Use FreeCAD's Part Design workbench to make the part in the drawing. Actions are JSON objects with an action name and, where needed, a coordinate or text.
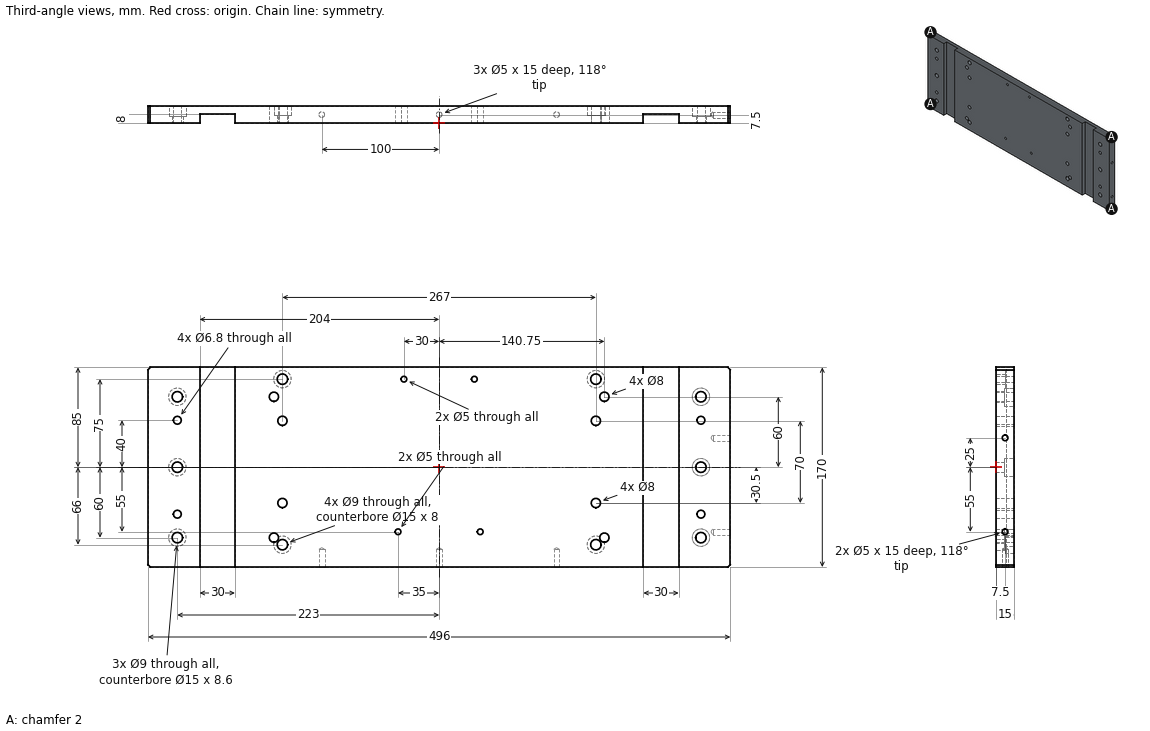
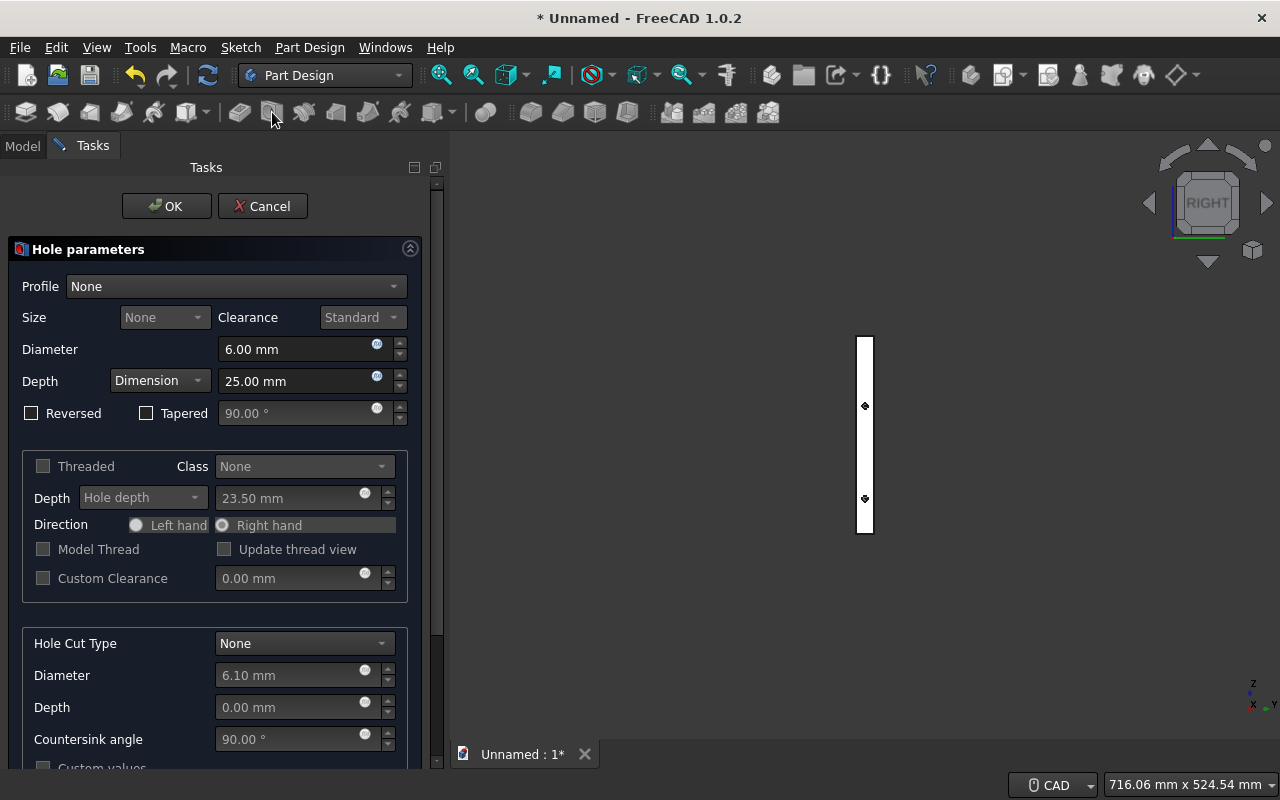
{"action": "triple_click", "coordinate": [305, 349]}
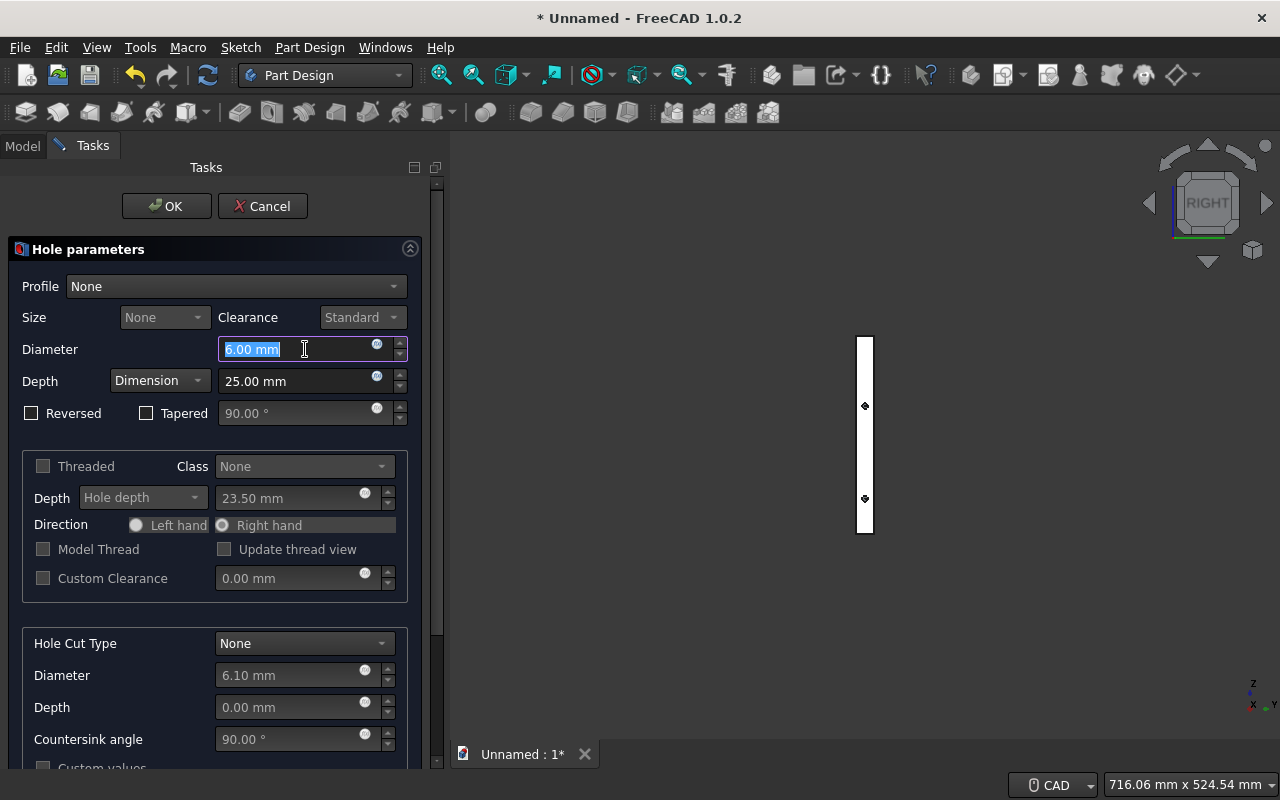
{"action": "type", "text": "5"}
{"action": "key", "text": "Tab"}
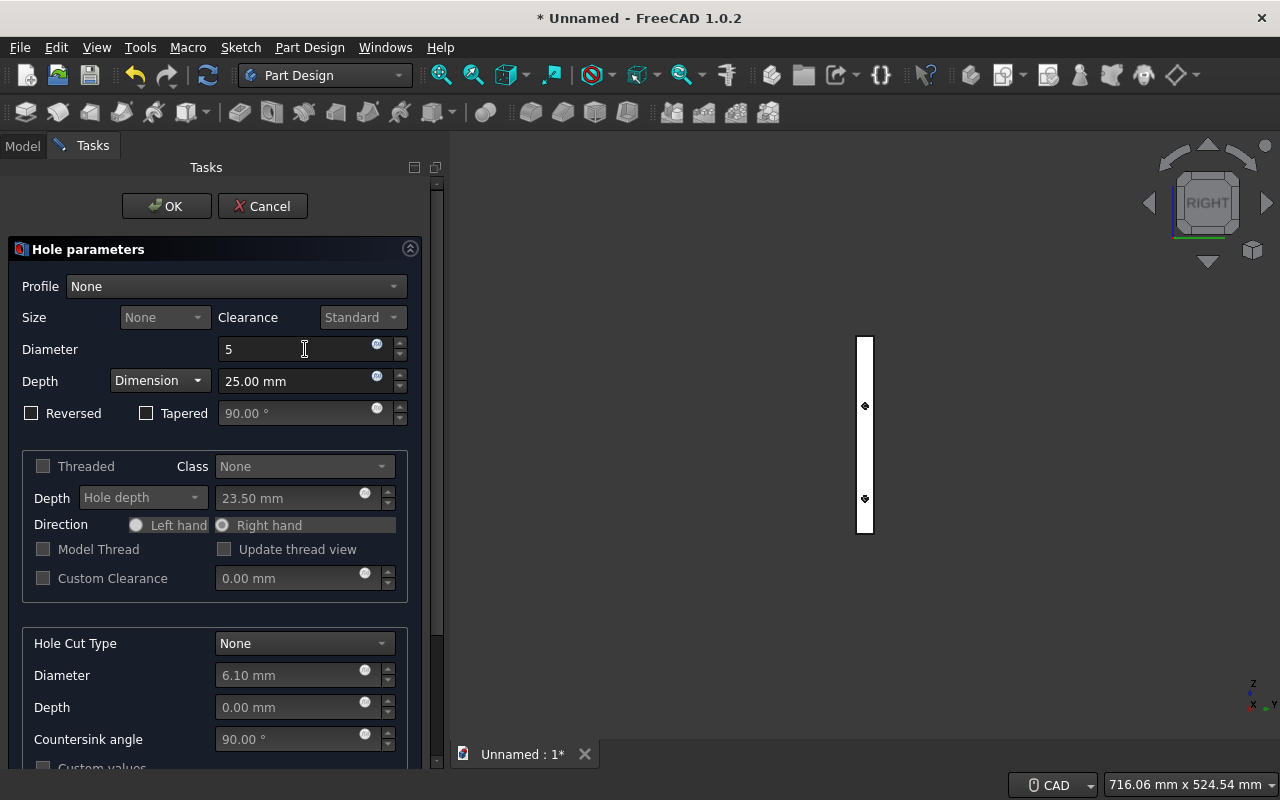
{"action": "left_click", "coordinate": [161, 380]}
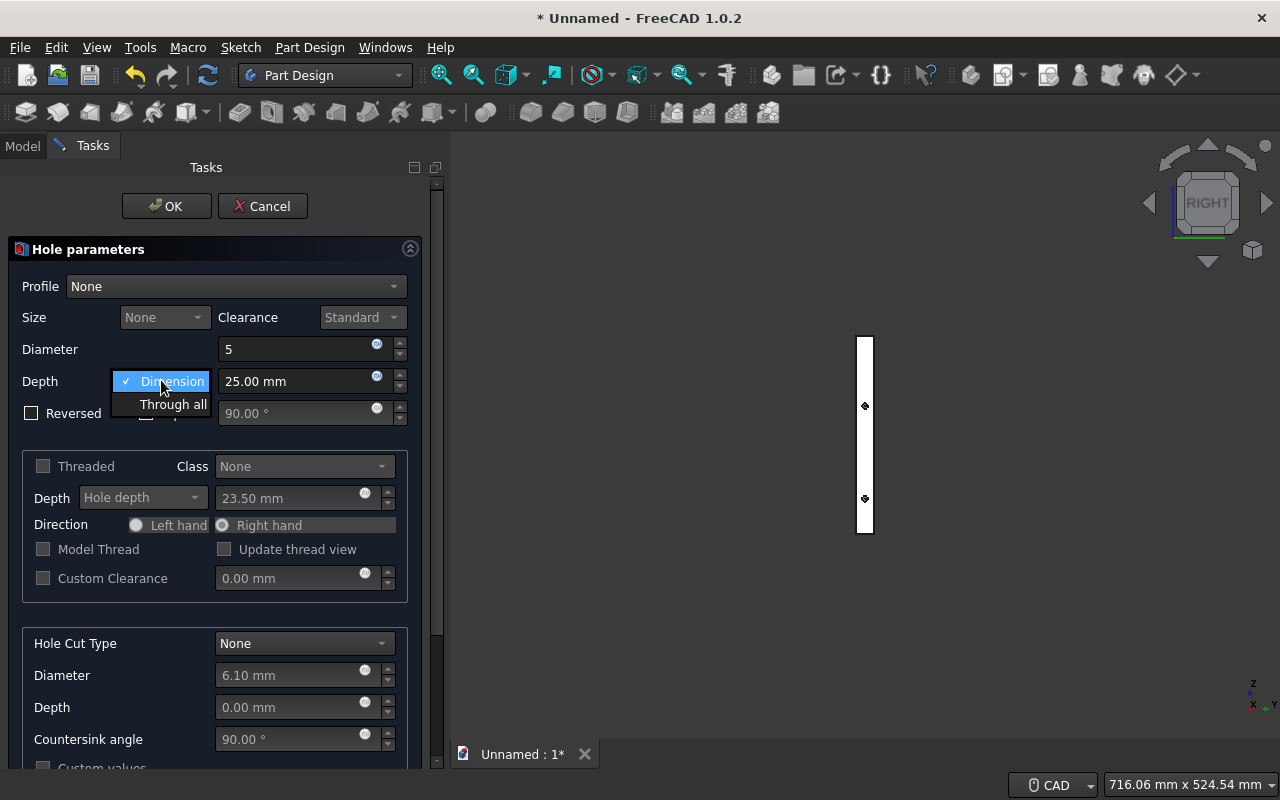
{"action": "left_click", "coordinate": [160, 404]}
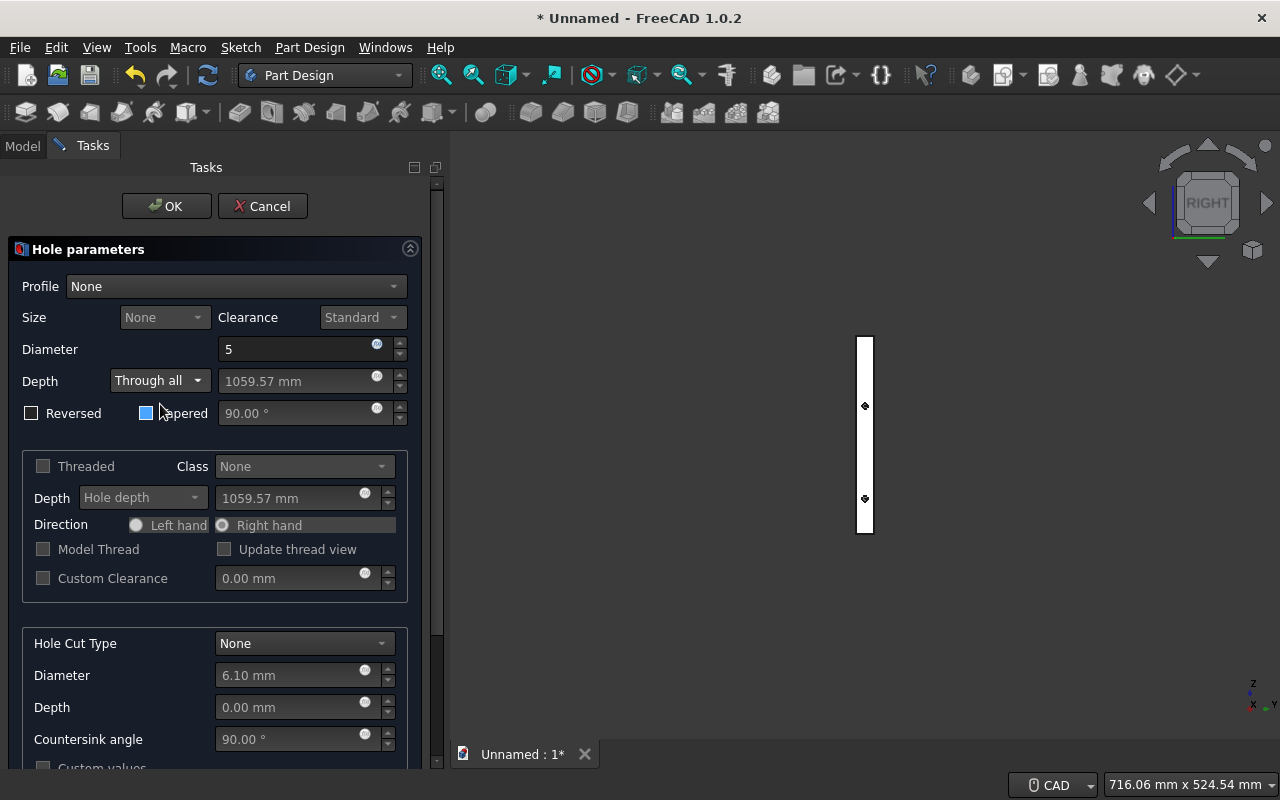
{"action": "left_click", "coordinate": [167, 206]}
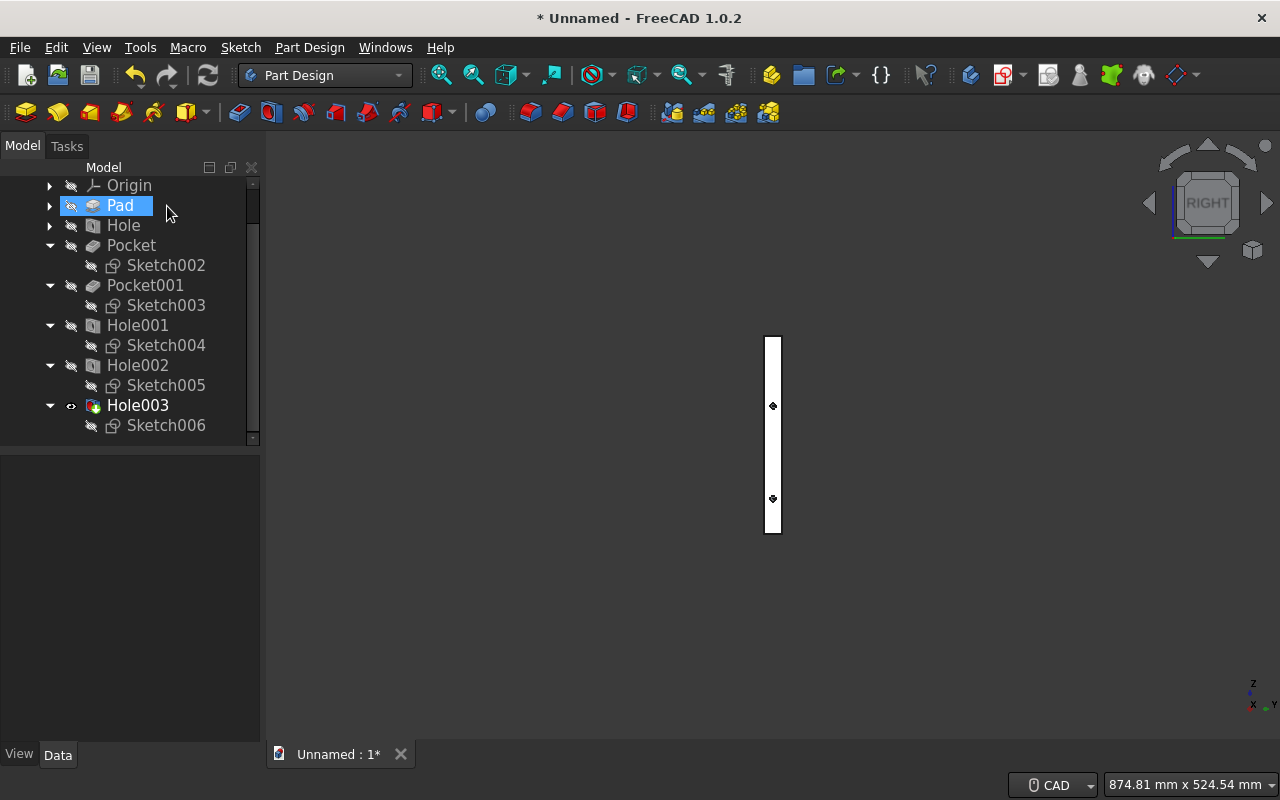
{"action": "left_click", "coordinate": [442, 76]}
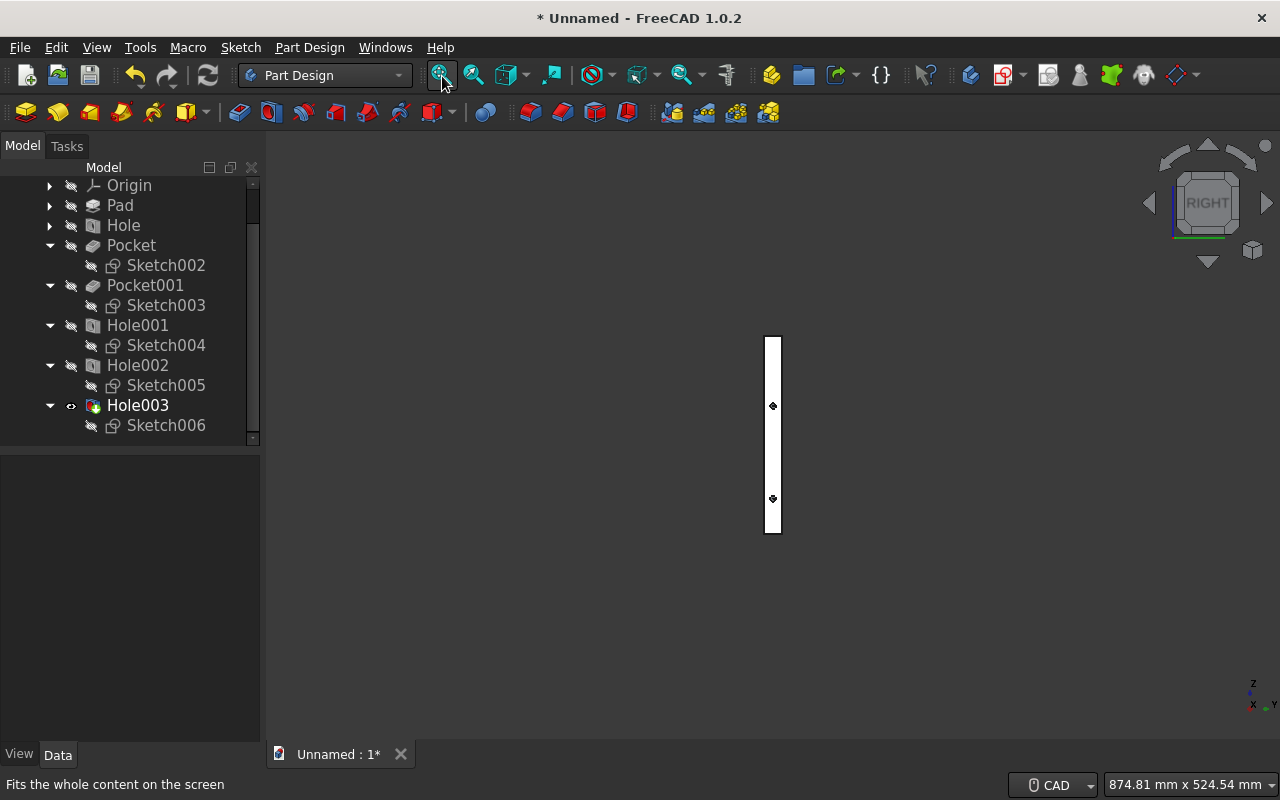
{"action": "left_click", "coordinate": [773, 533]}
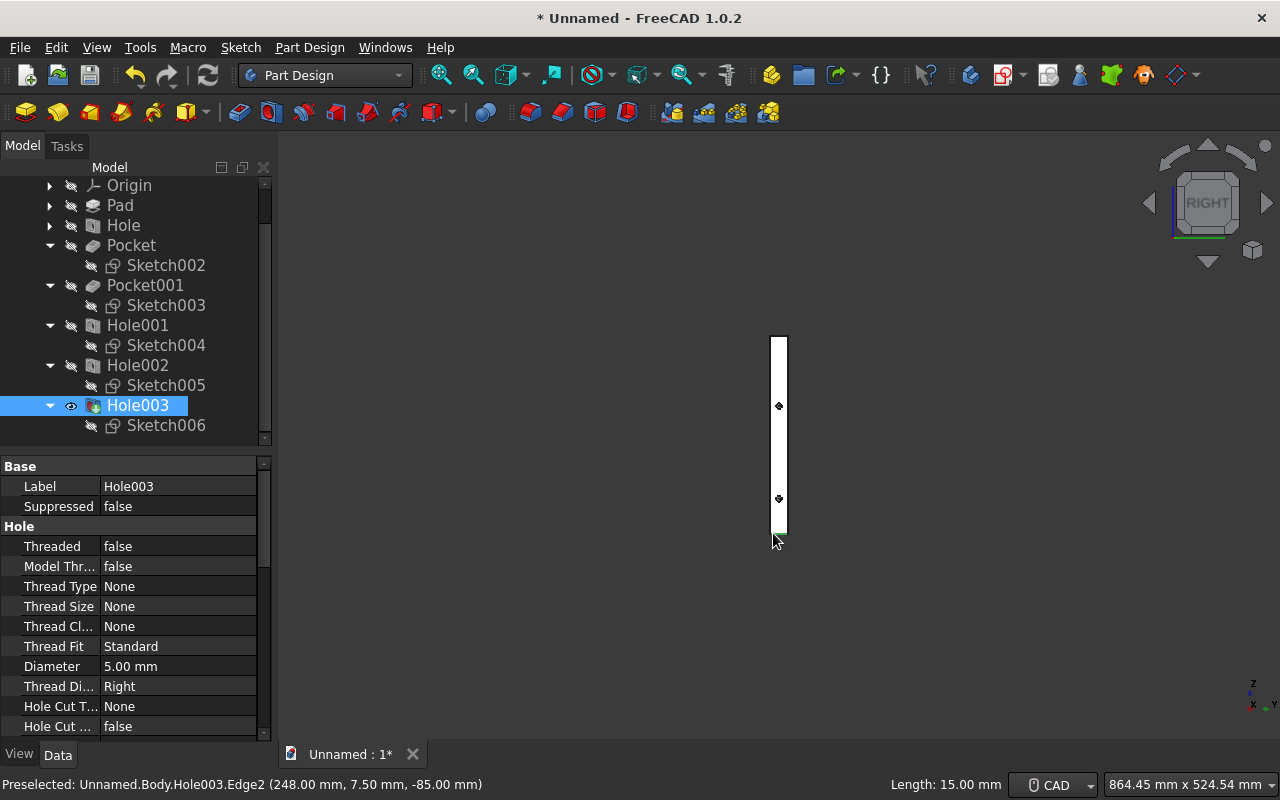
{"action": "scroll", "coordinate": [779, 335], "scroll_direction": "up", "scroll_amount": 5}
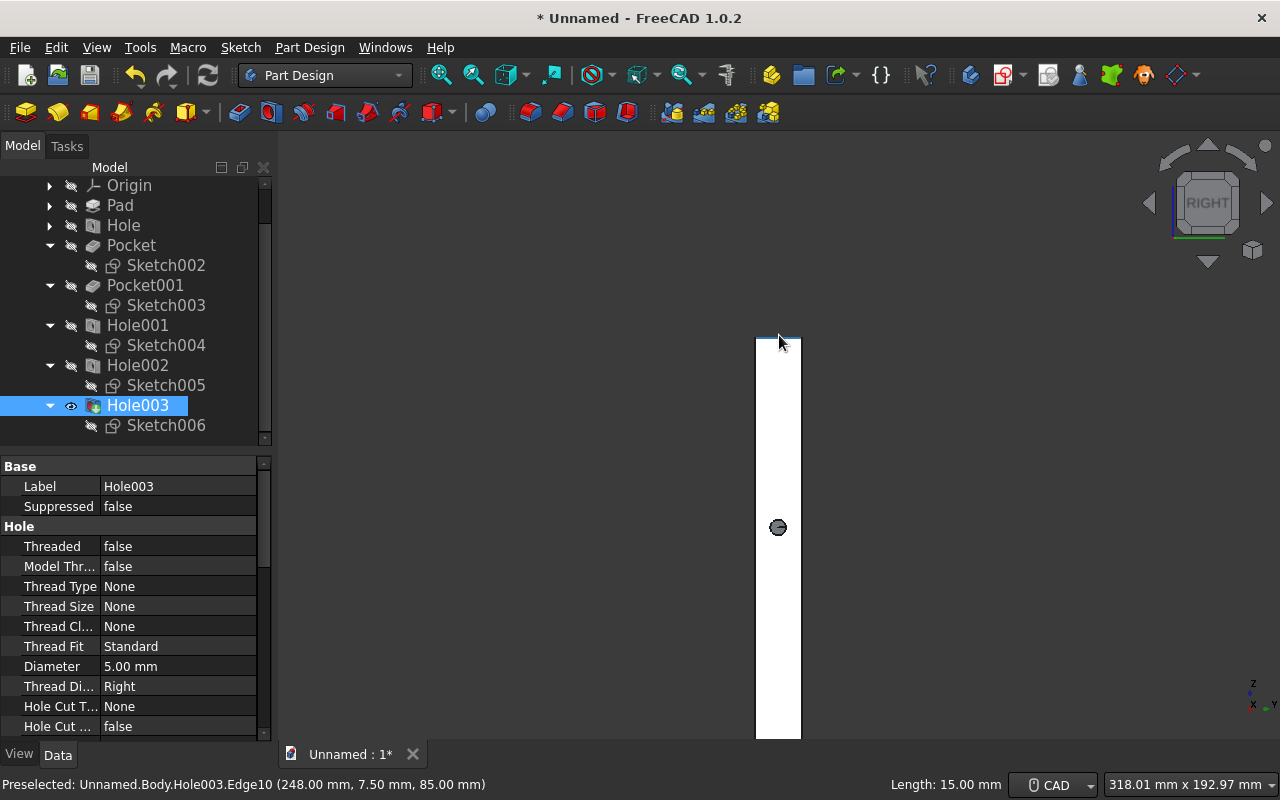
{"action": "left_click", "coordinate": [442, 76]}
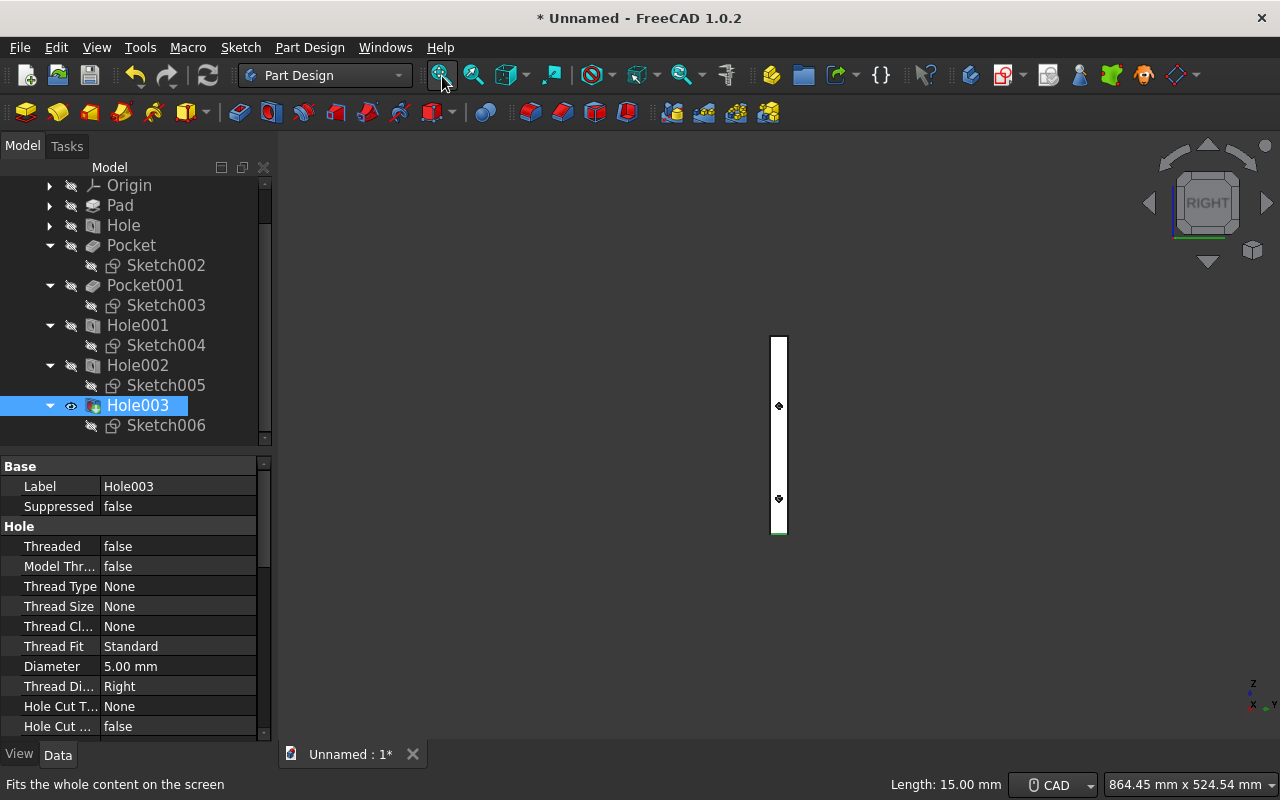
{"action": "key", "text": "0"}